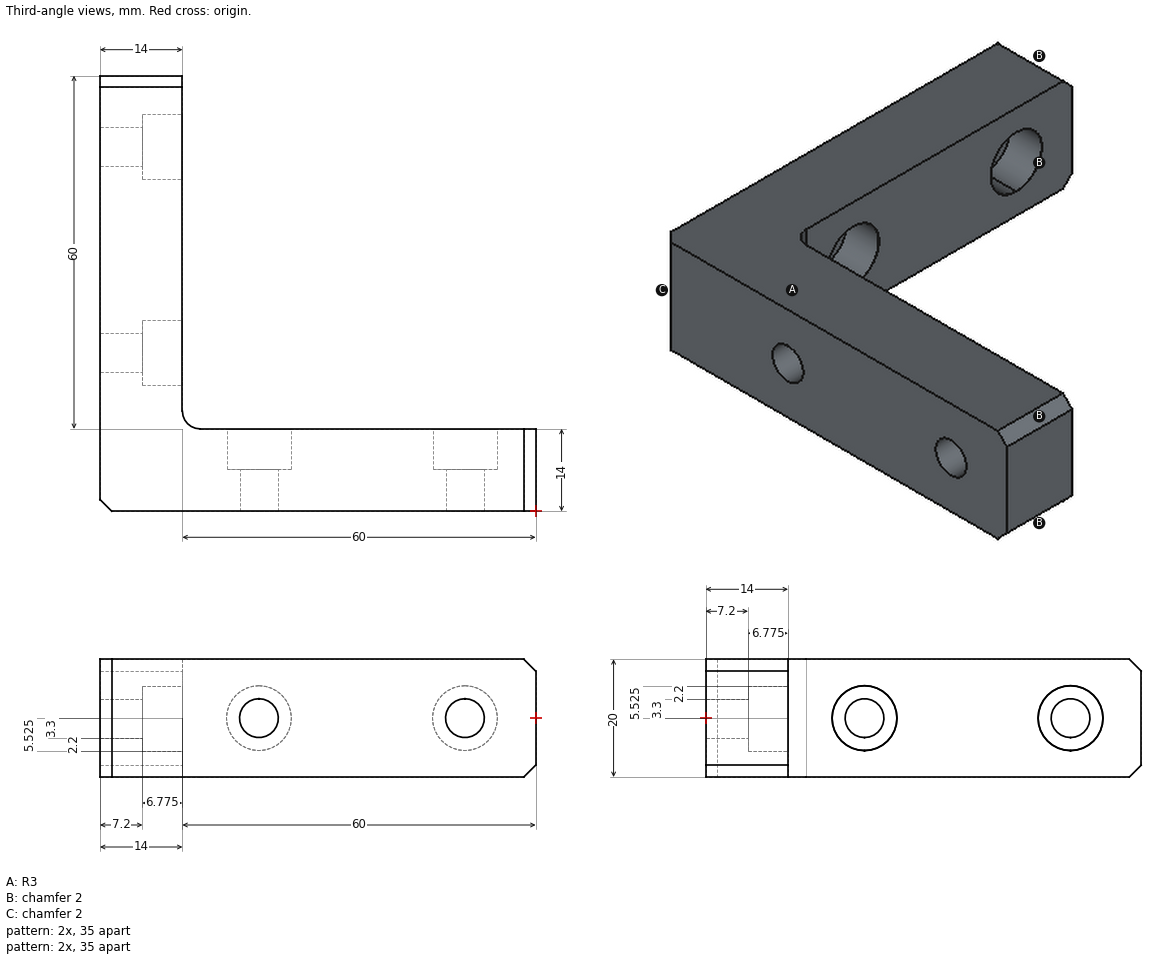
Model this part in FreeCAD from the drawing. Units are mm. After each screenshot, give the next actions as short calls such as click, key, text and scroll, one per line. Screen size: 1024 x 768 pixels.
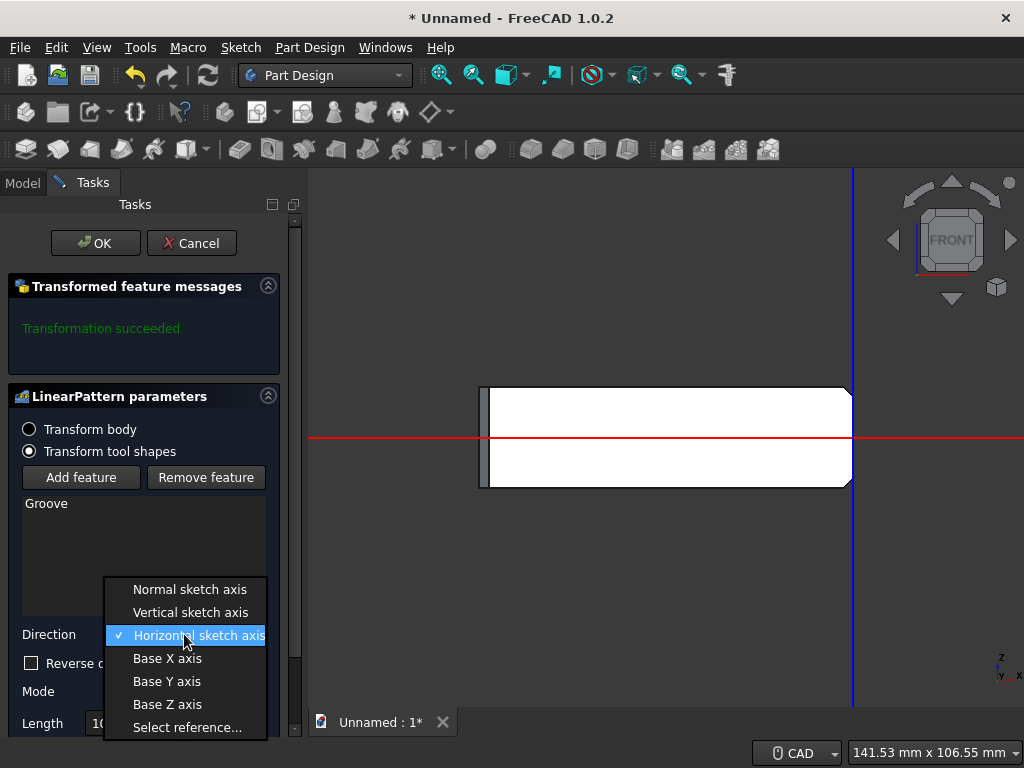
click(184, 682)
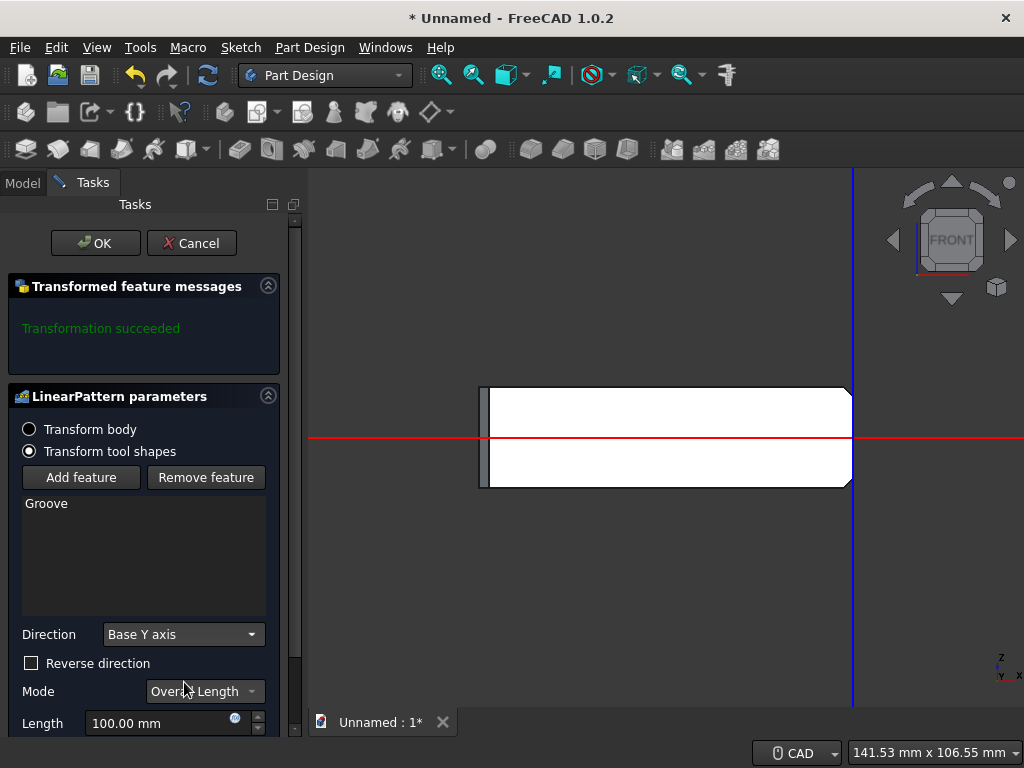
click(206, 692)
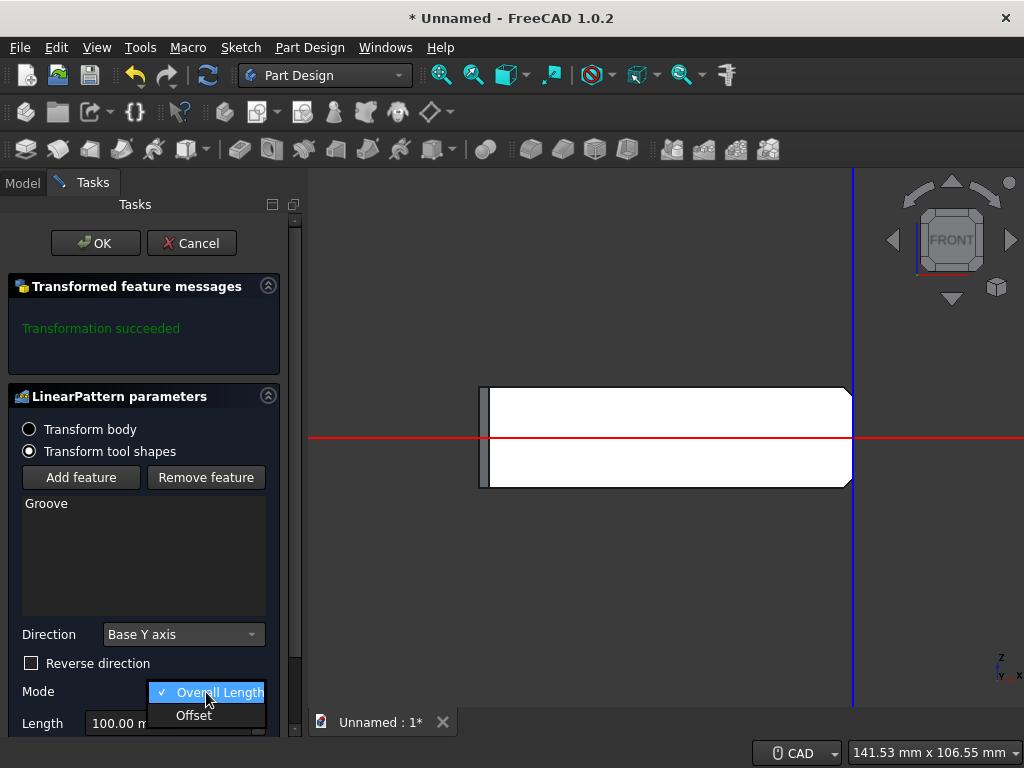
click(206, 716)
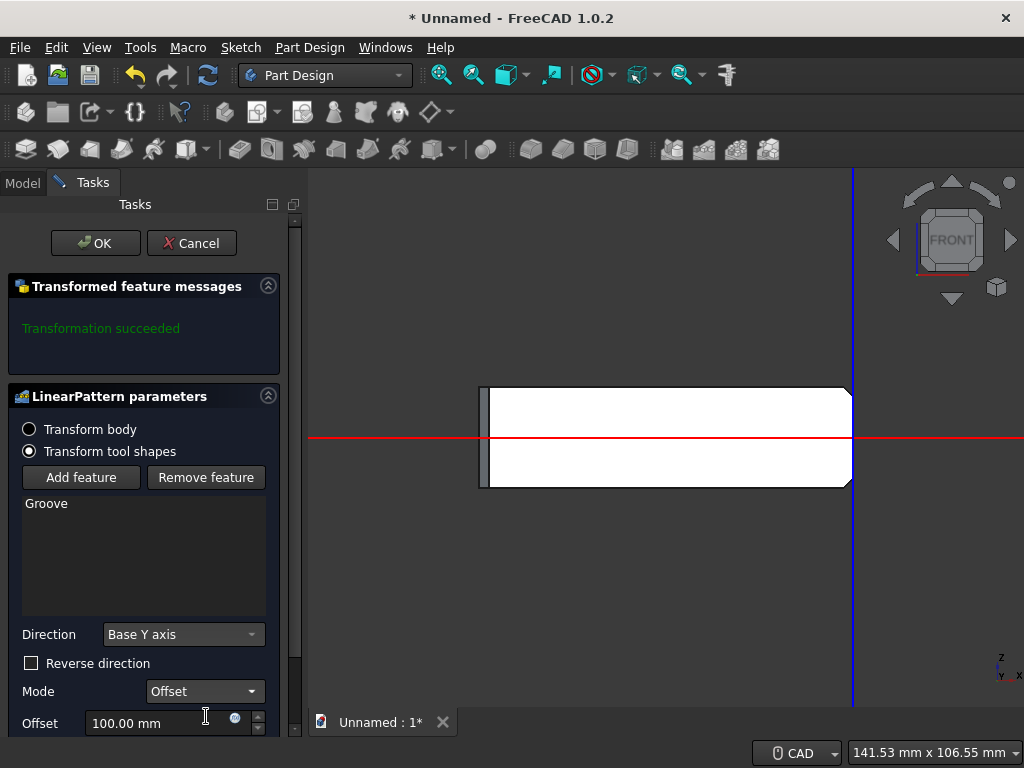
triple_click(168, 723)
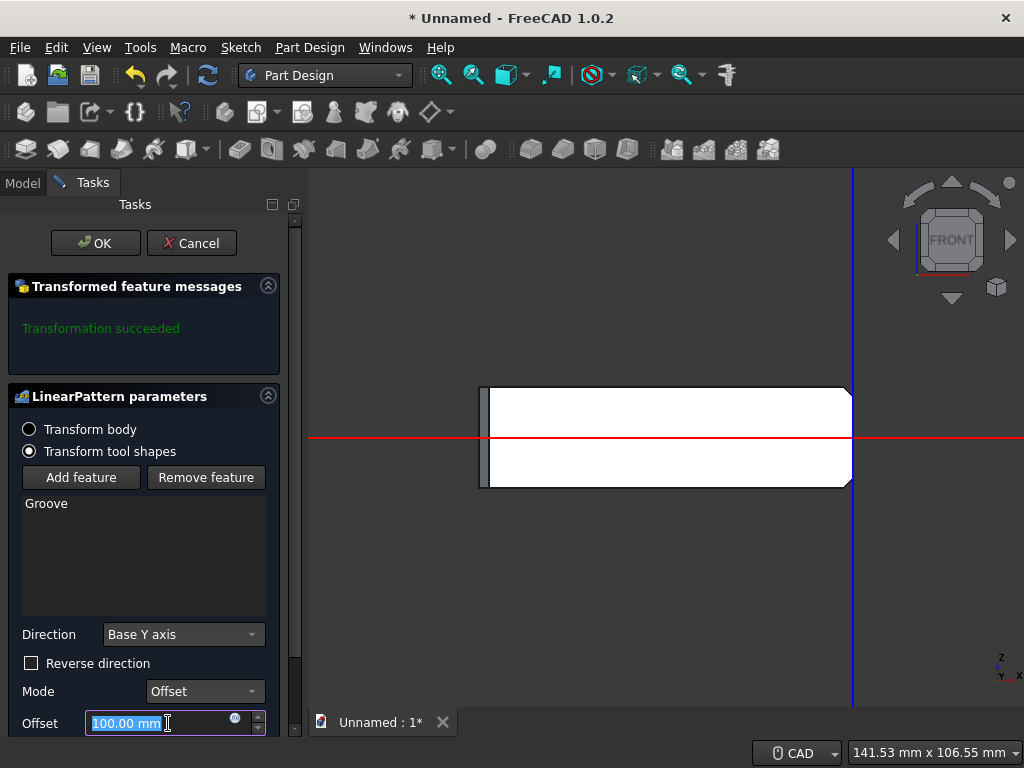
text(35)
key(Tab)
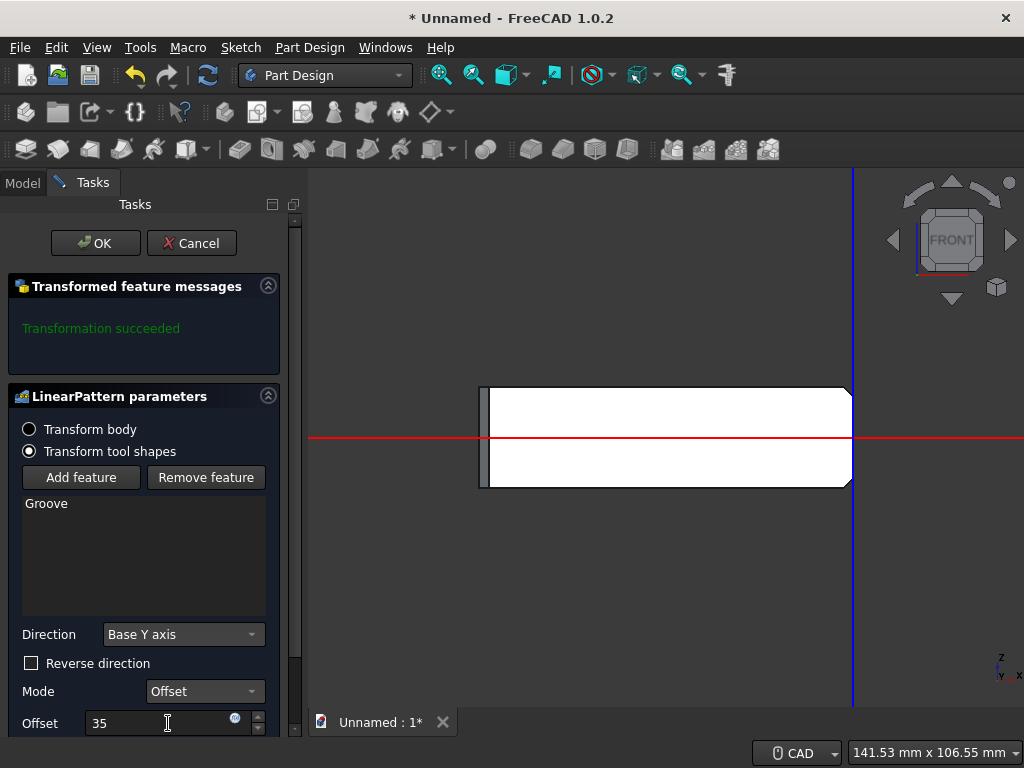
scroll(295, 475, down, 2)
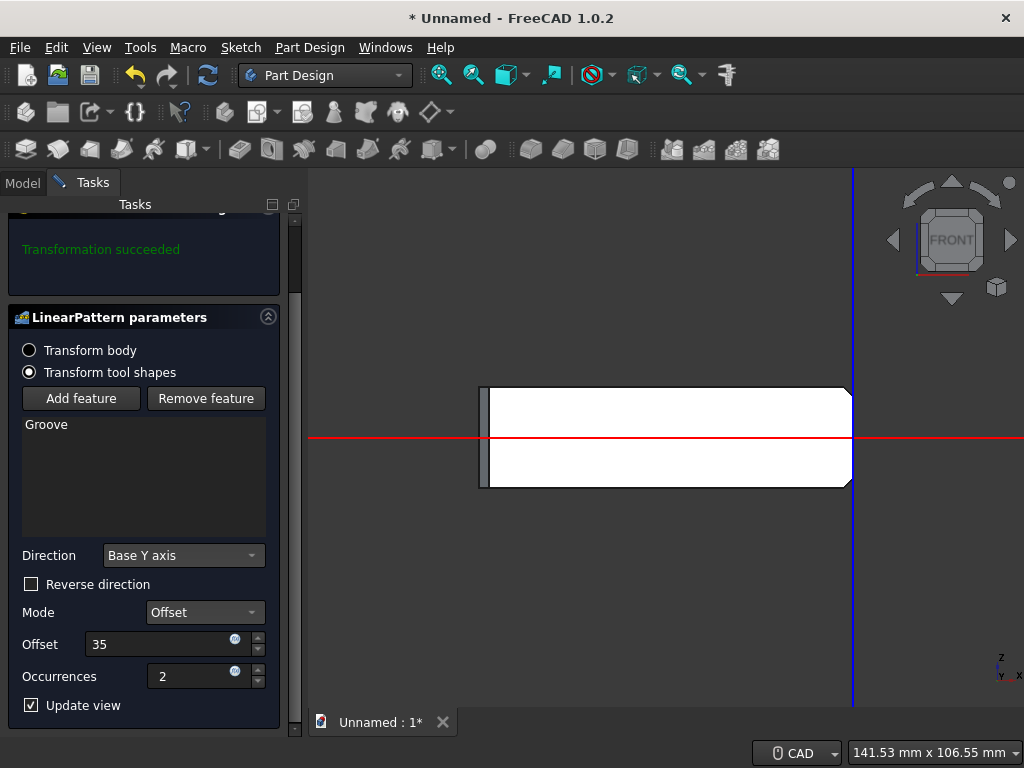
triple_click(198, 676)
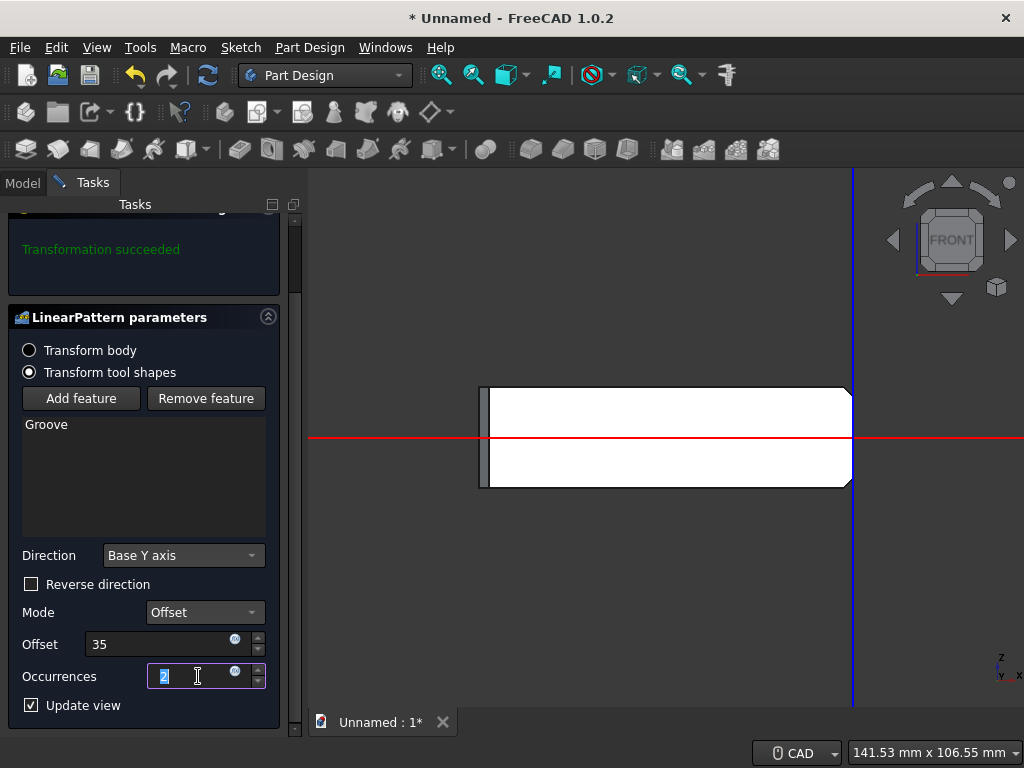
text(2)
key(Tab)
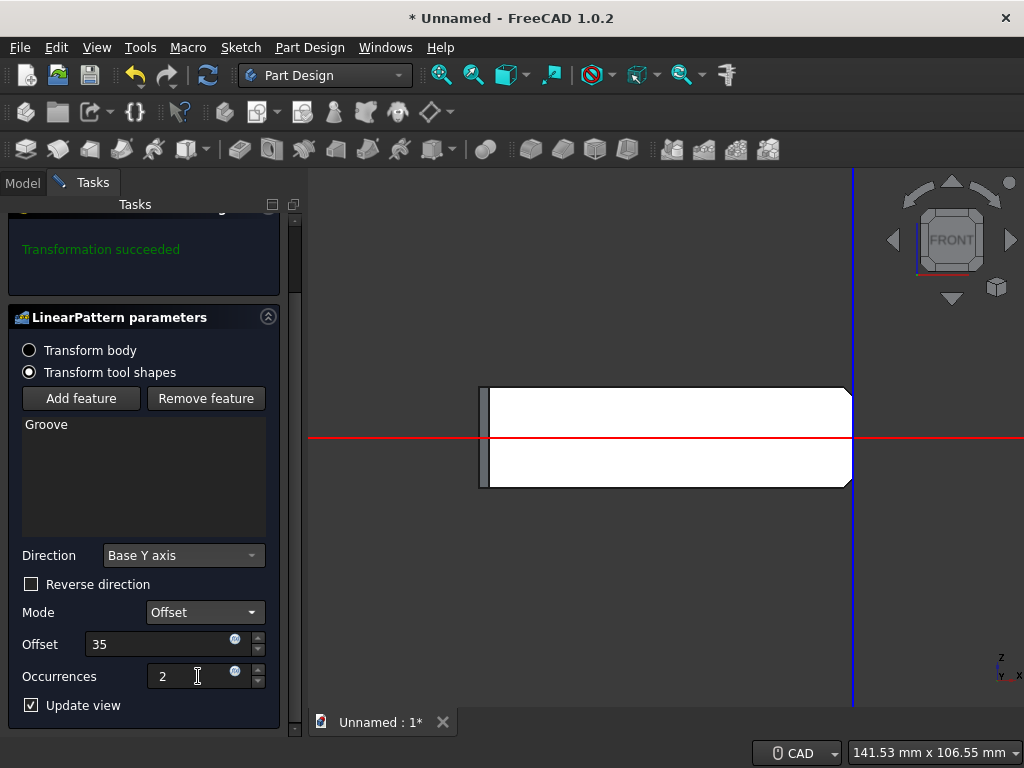
click(30, 584)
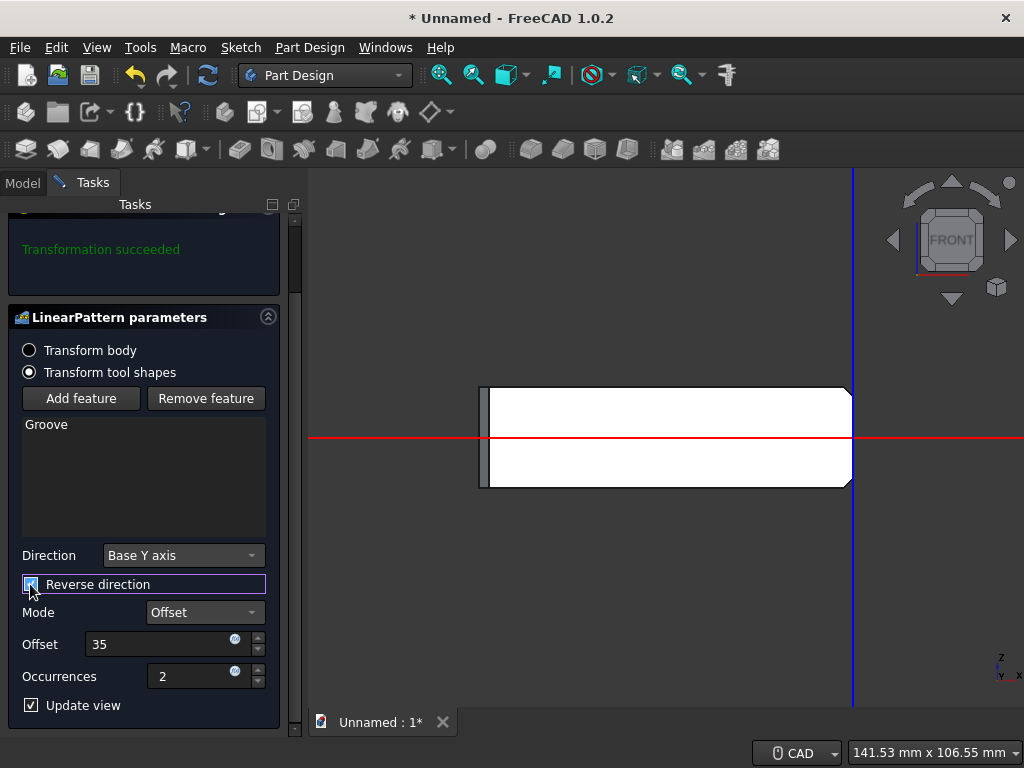
scroll(295, 475, up, 3)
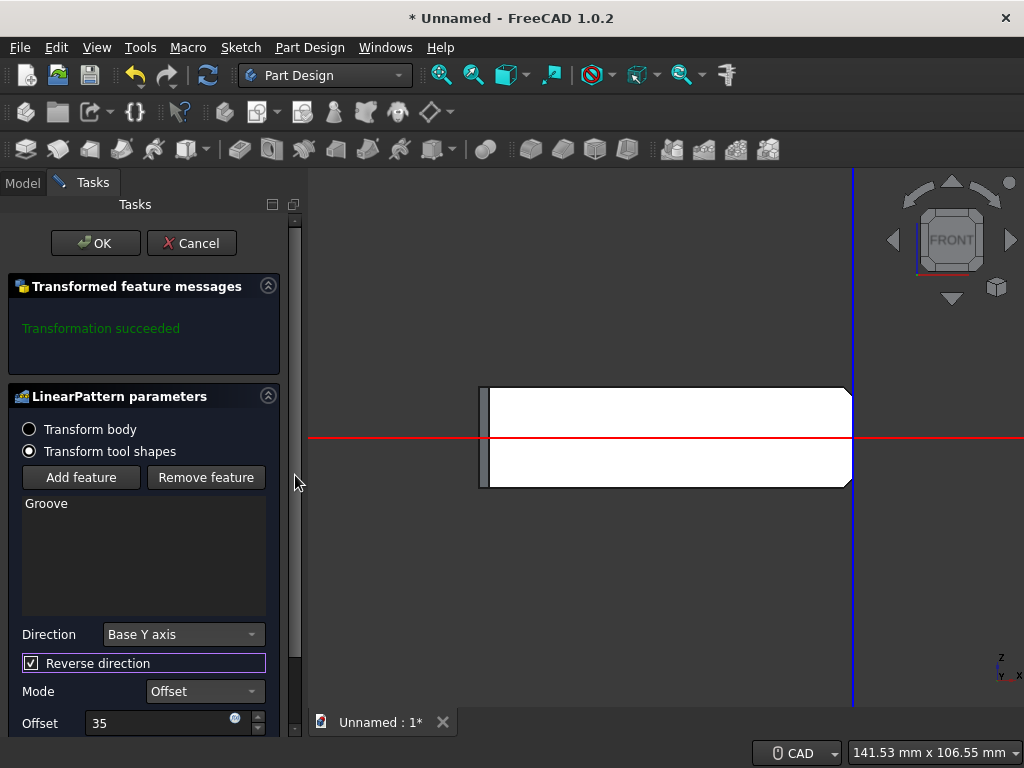
click(96, 243)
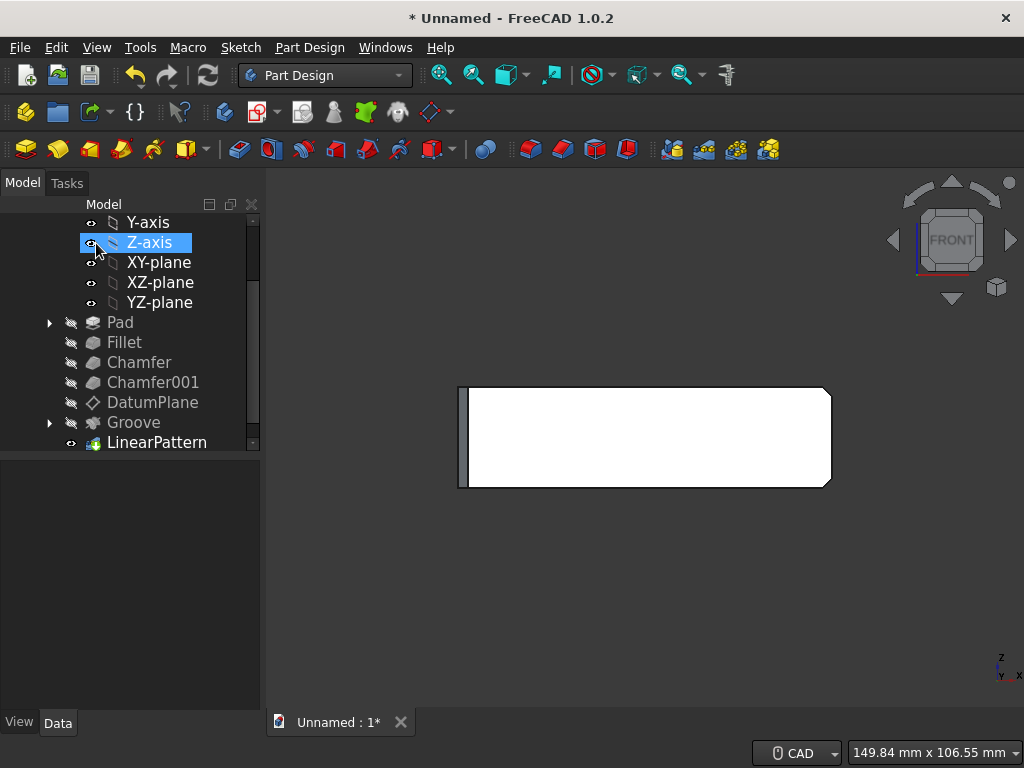
scroll(160, 338, down, 3)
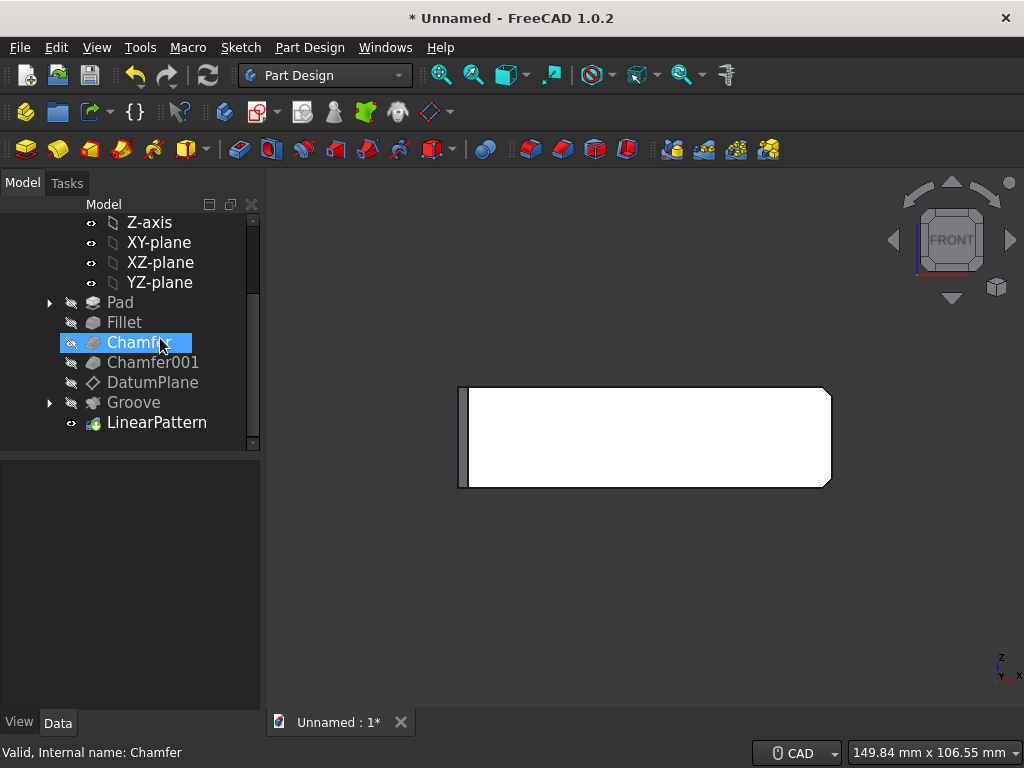
scroll(160, 318, up, 15)